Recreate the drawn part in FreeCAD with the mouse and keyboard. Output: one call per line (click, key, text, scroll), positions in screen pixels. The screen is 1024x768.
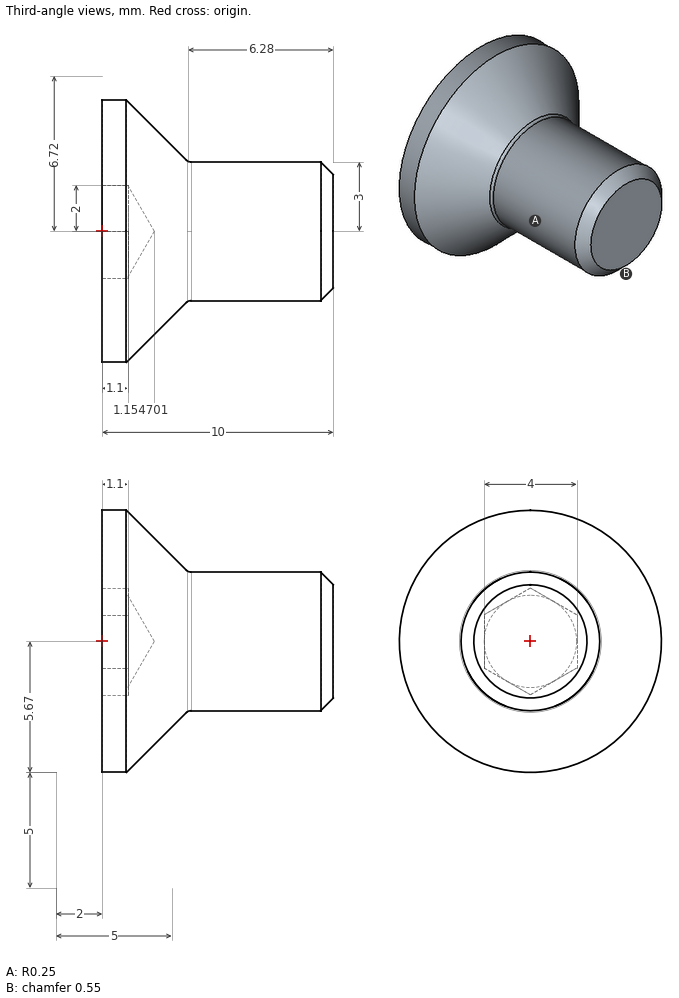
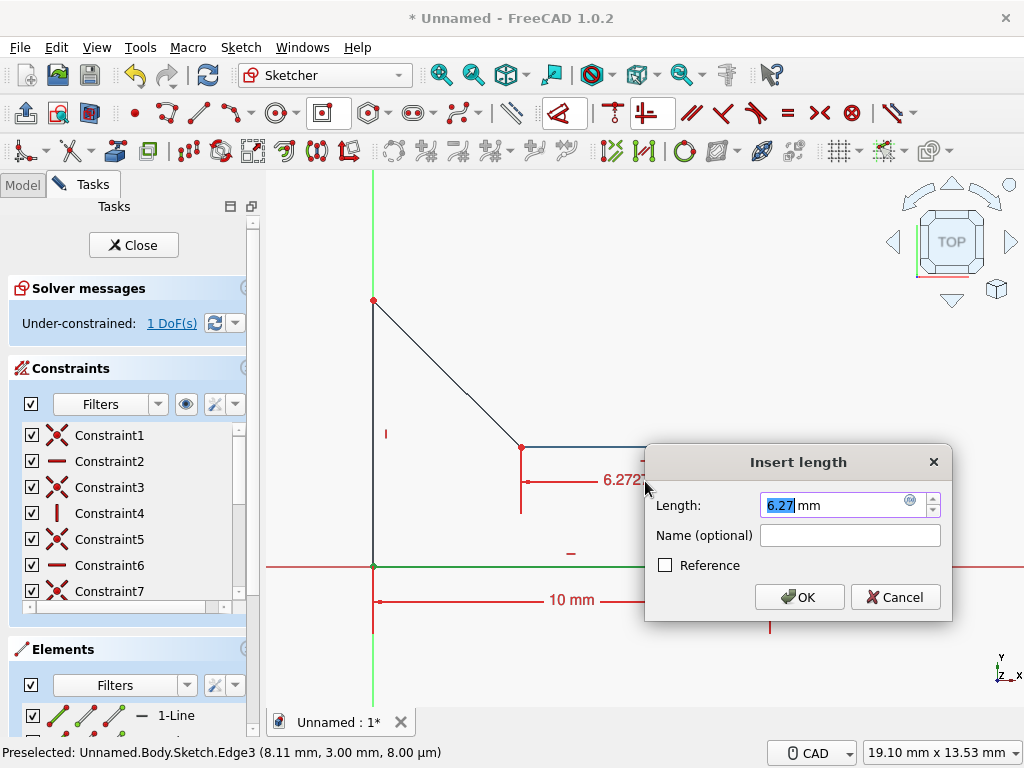
text(6.28)
key(Return)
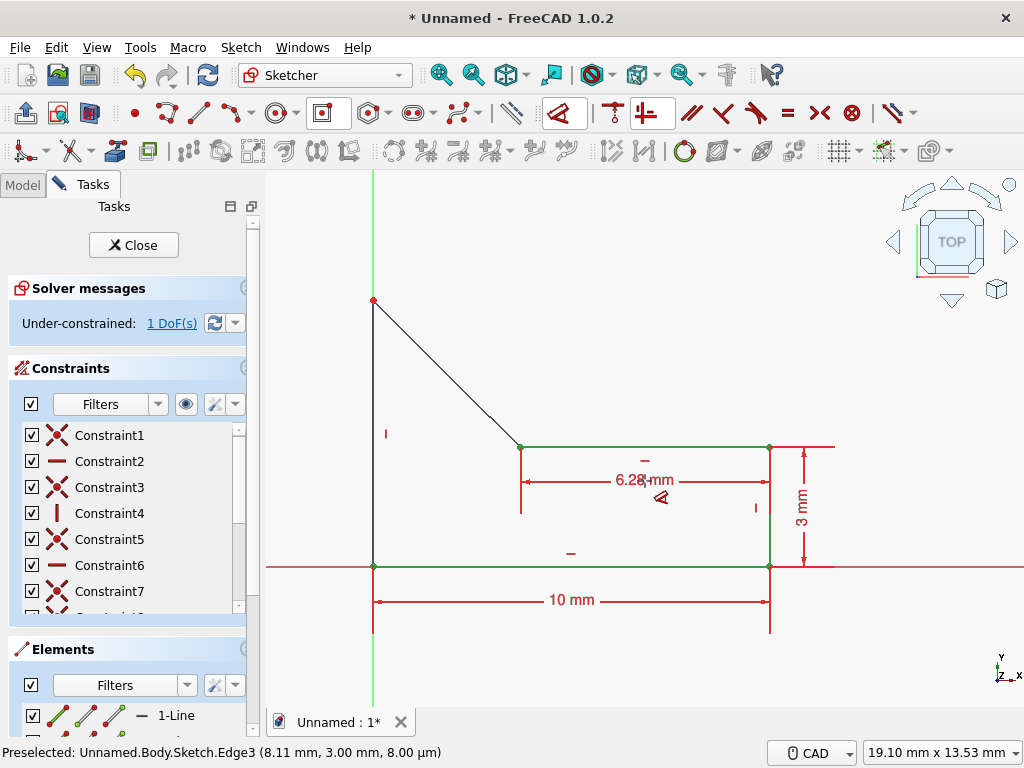
click(373, 381)
click(339, 434)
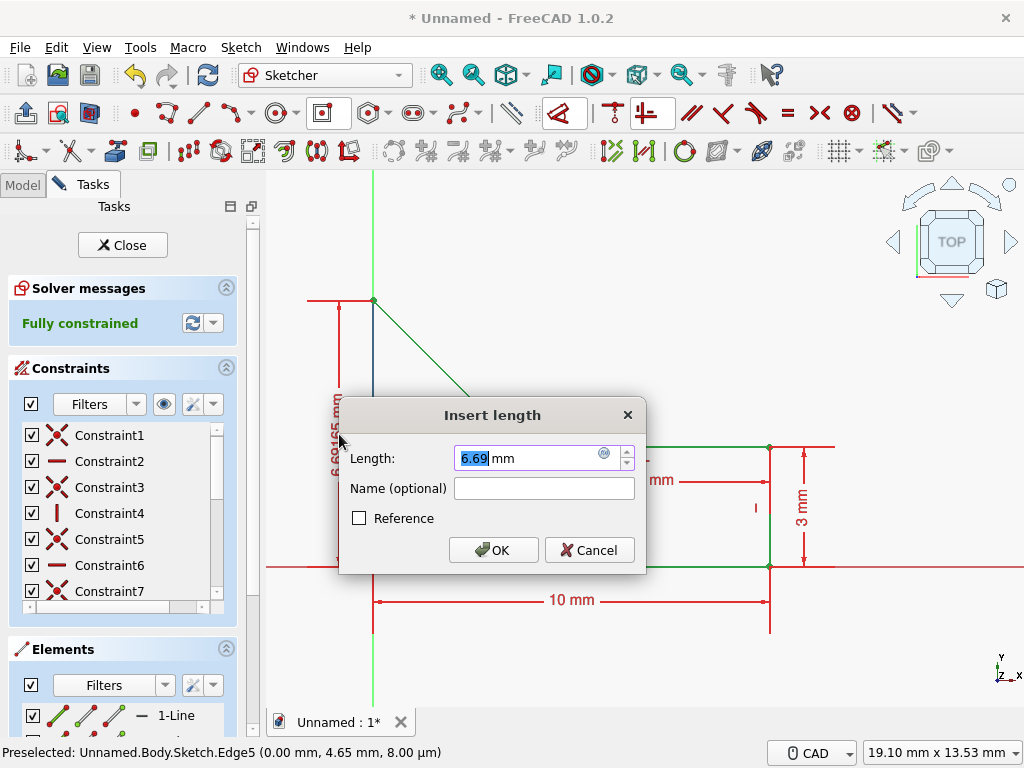
text(6.72)
key(Return)
key(Escape)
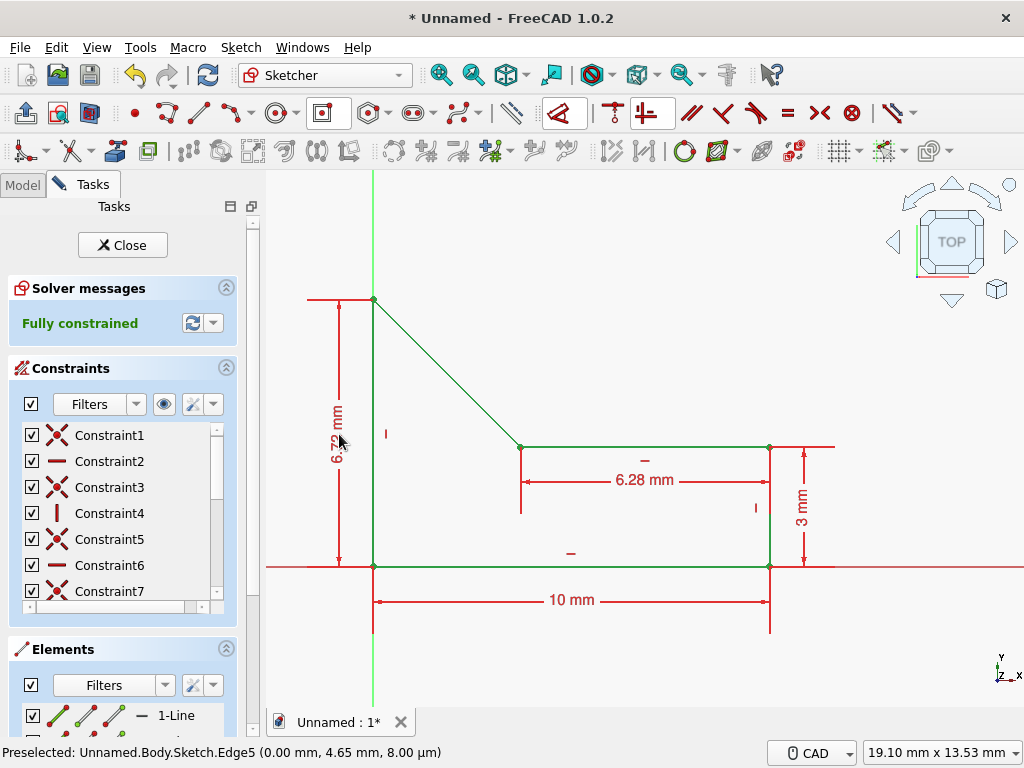
click(123, 245)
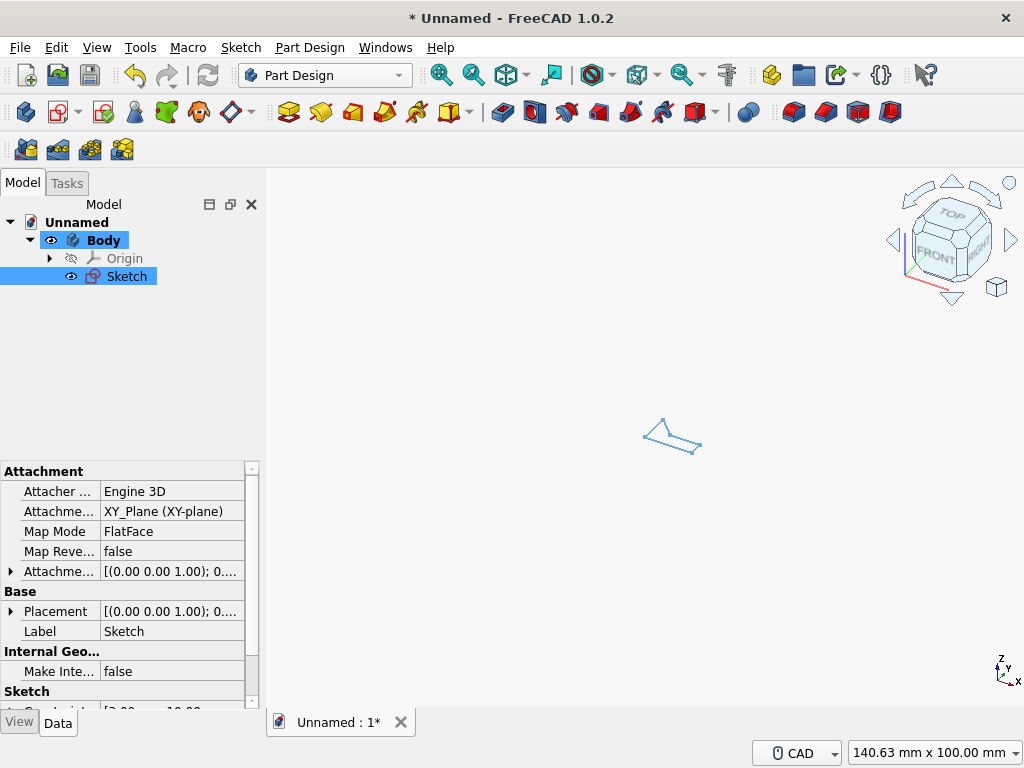
click(322, 112)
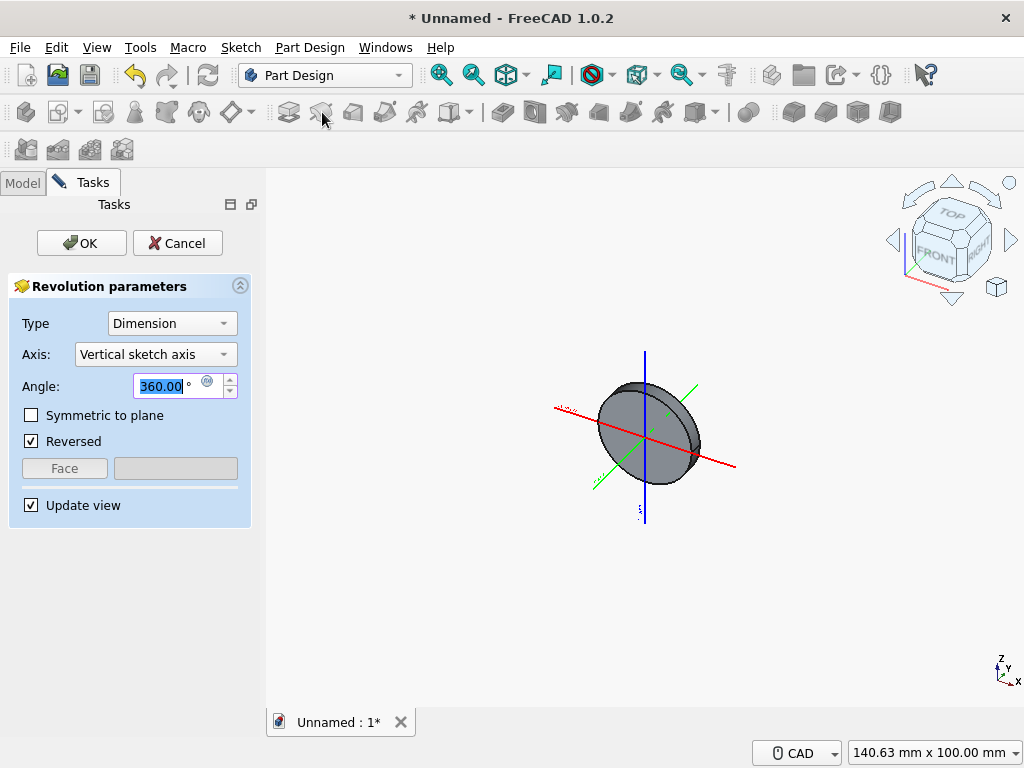
click(156, 354)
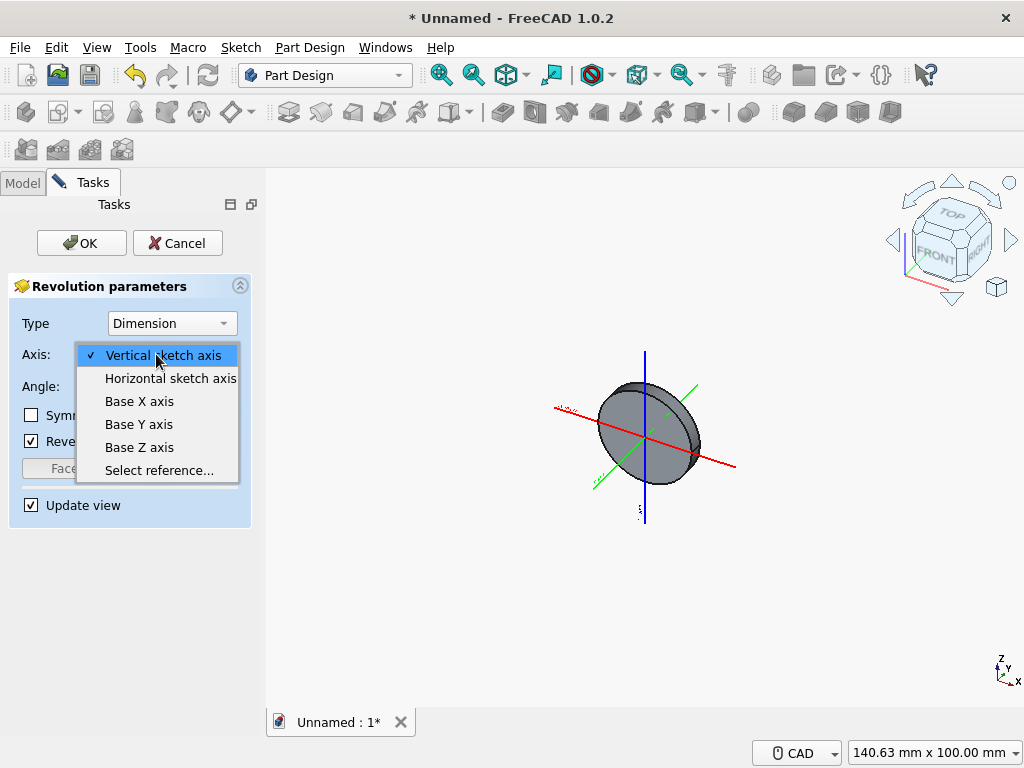
click(156, 378)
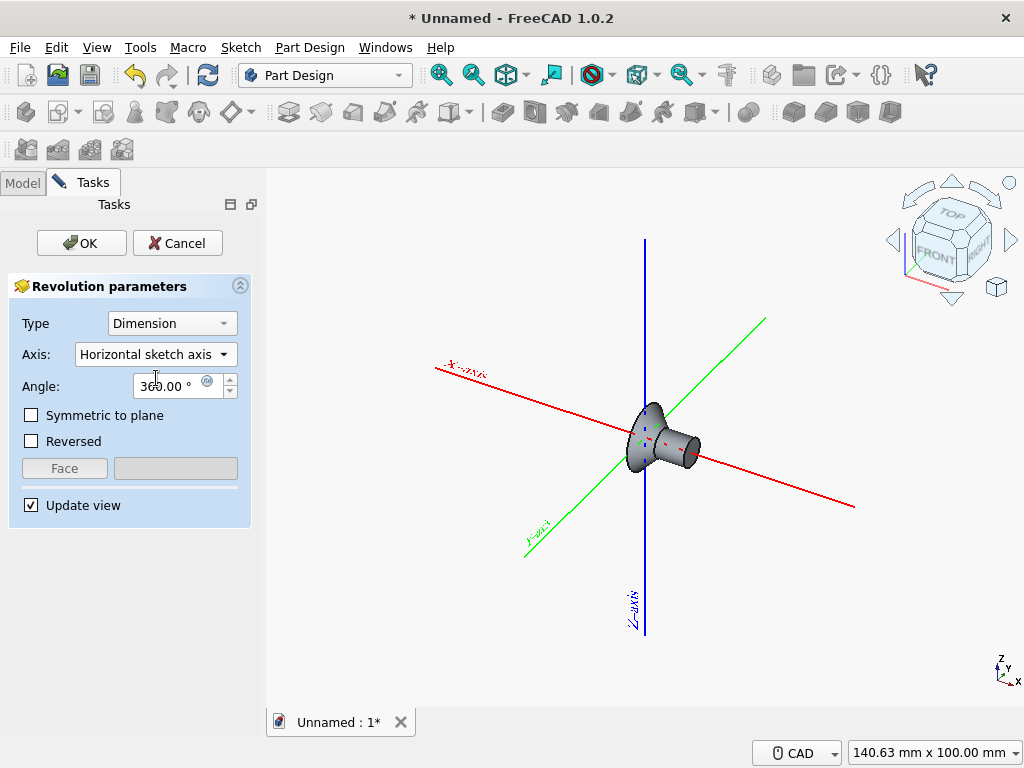
click(82, 243)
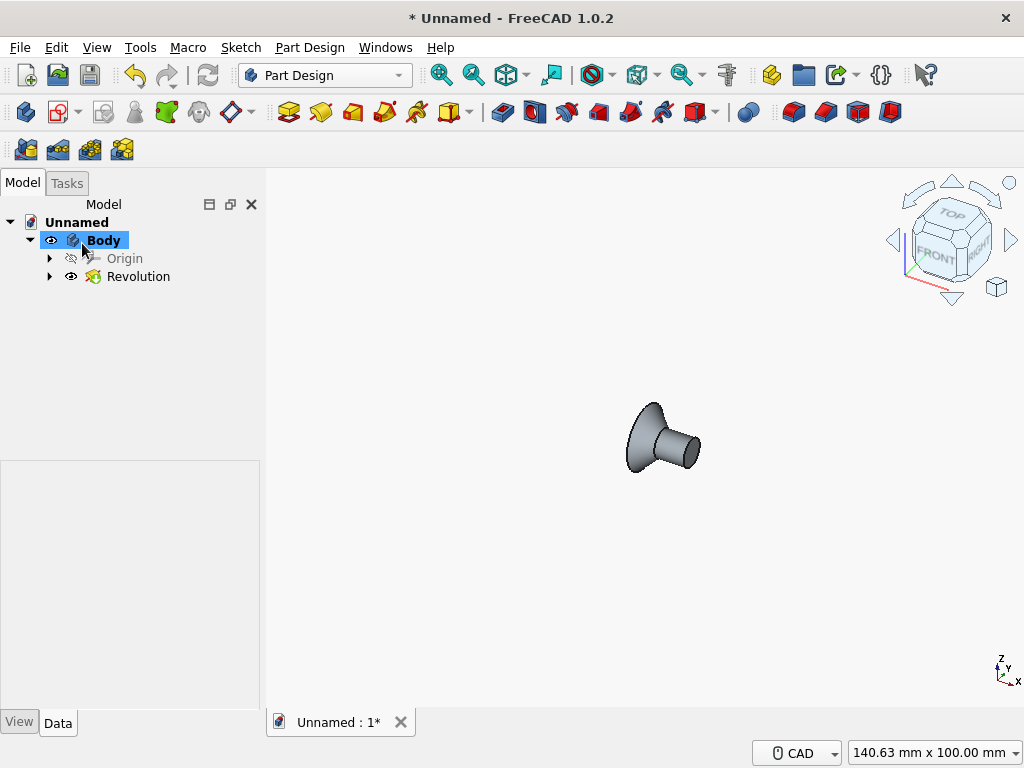
key(v)
key(f)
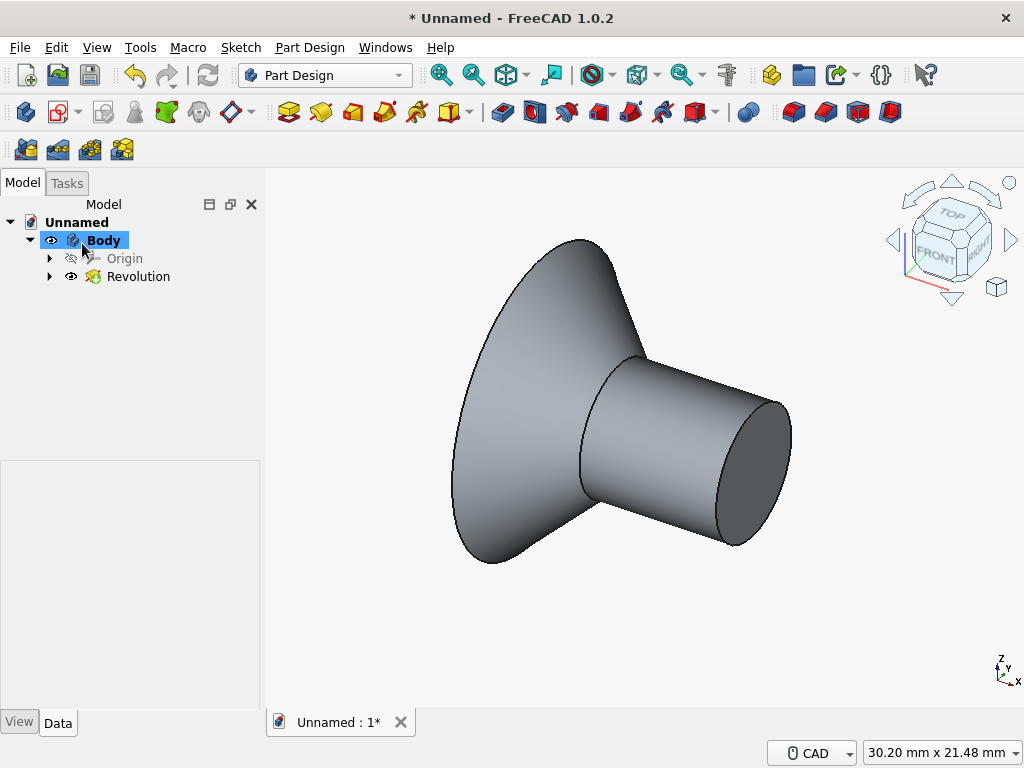
key(6)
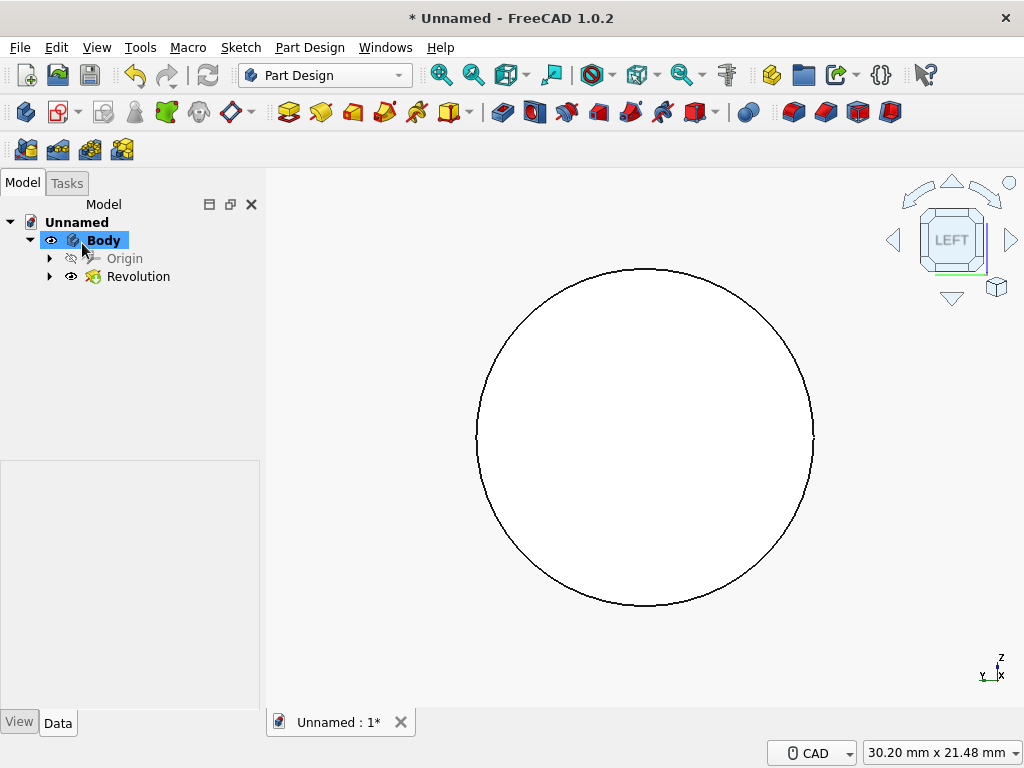
click(645, 436)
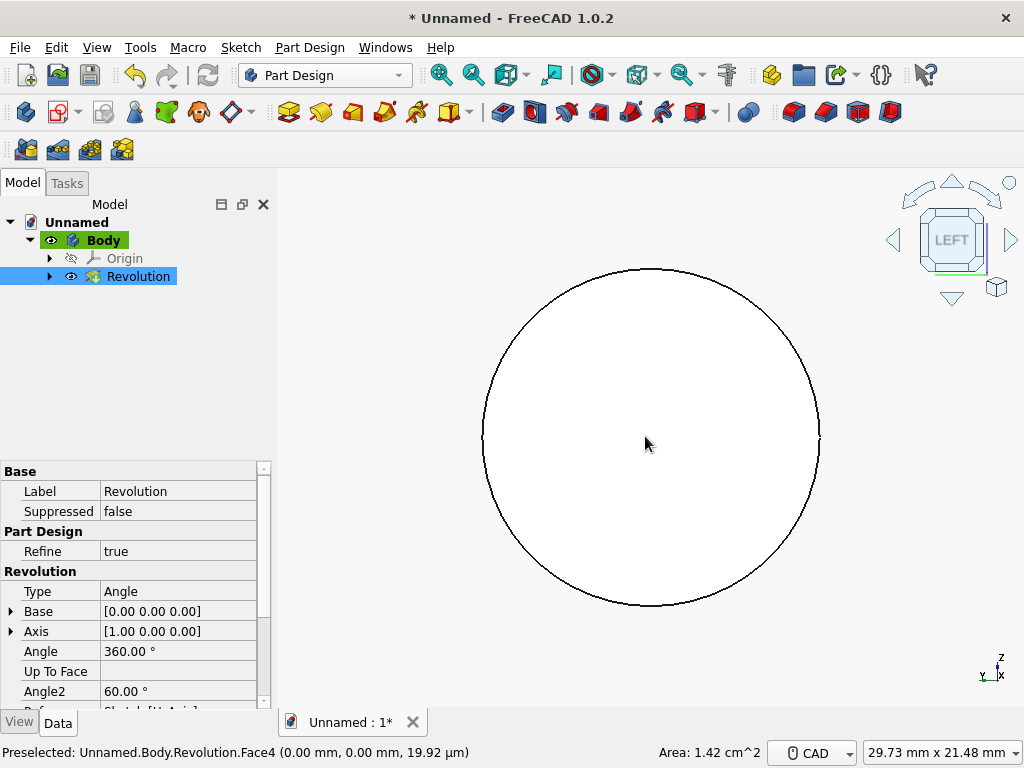
click(58, 112)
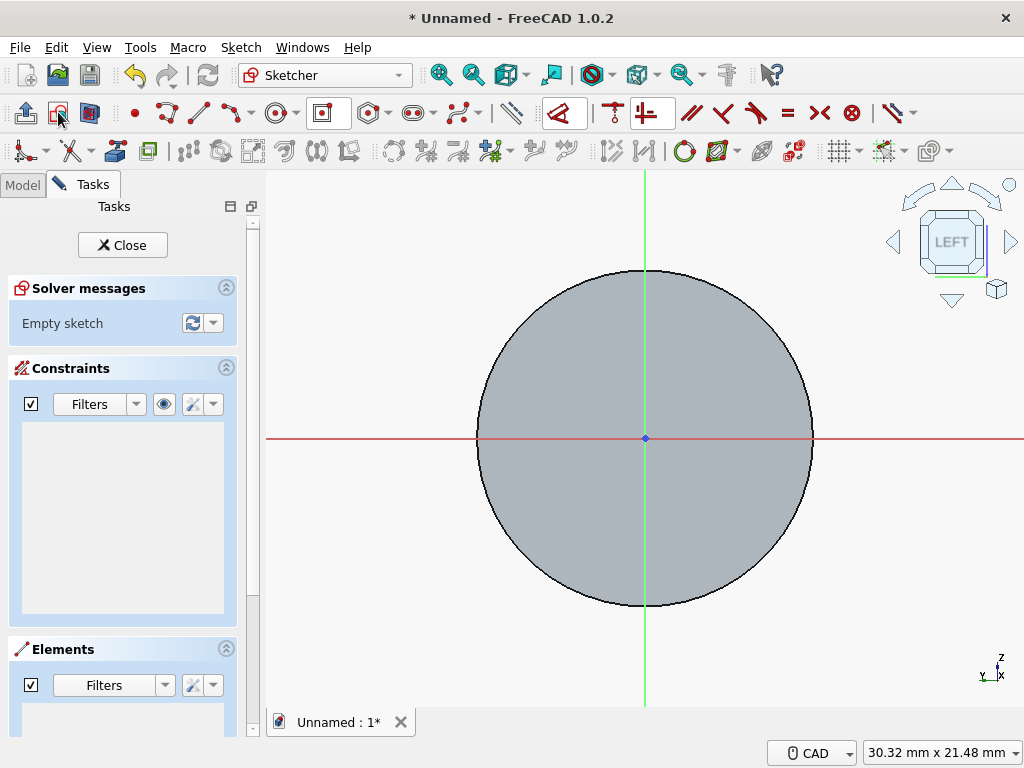
scroll(685, 439, up, 5)